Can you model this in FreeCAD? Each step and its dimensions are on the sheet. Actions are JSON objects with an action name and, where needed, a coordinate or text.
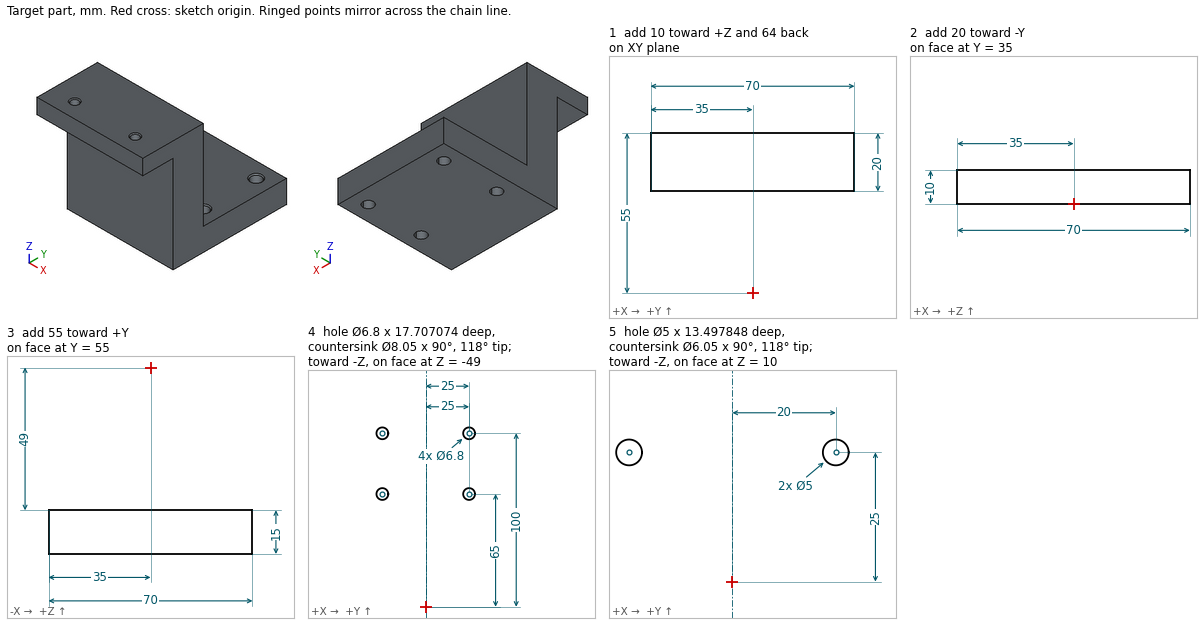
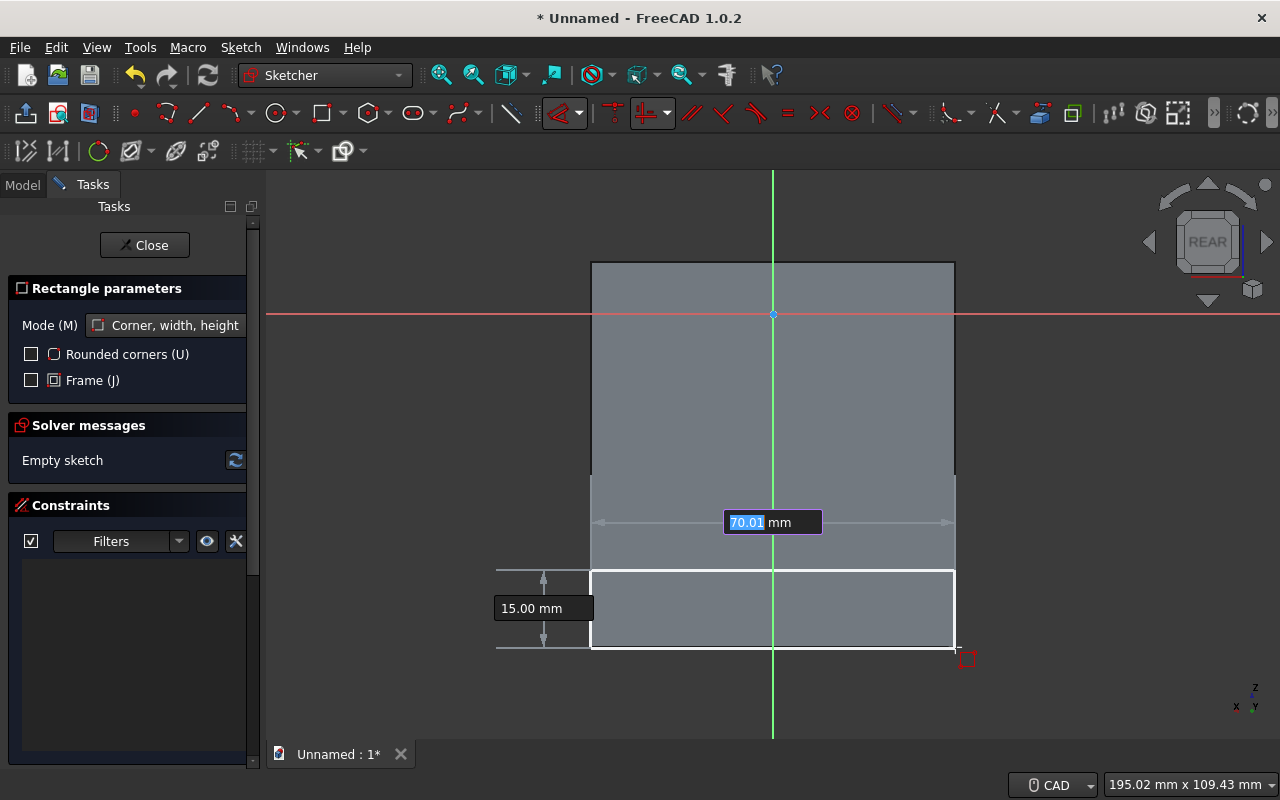
{"action": "type", "text": "70"}
{"action": "key", "text": "Tab"}
{"action": "type", "text": "15"}
{"action": "key", "text": "Return"}
{"action": "key", "text": "Escape"}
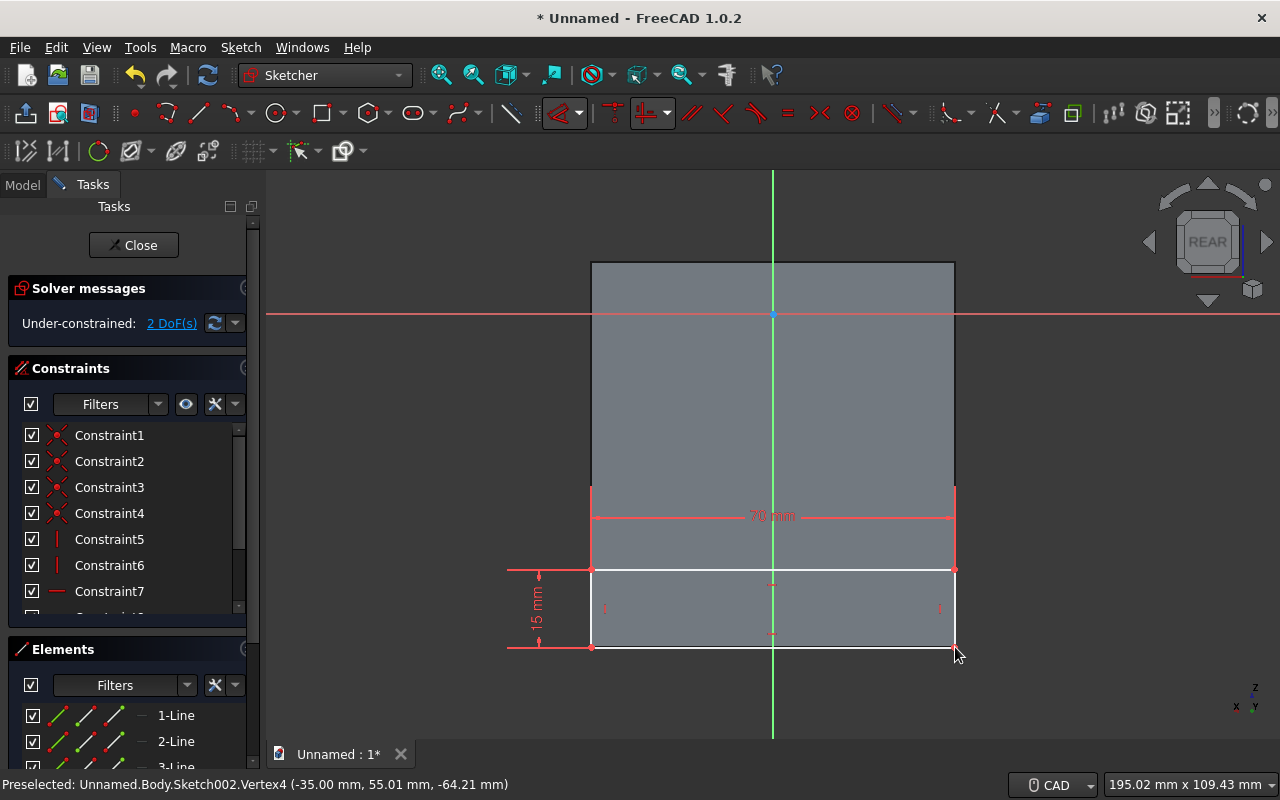
{"action": "left_click", "coordinate": [591, 570]}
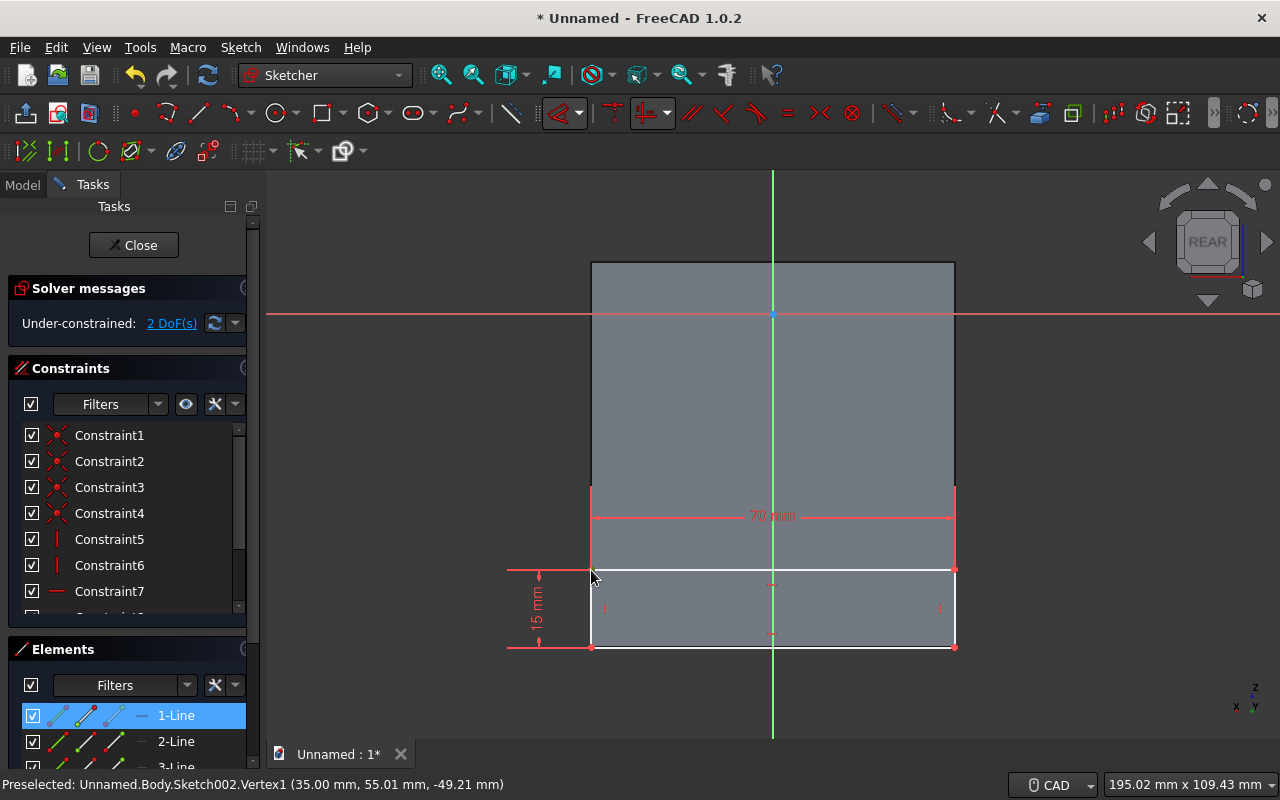
{"action": "left_click", "coordinate": [582, 114]}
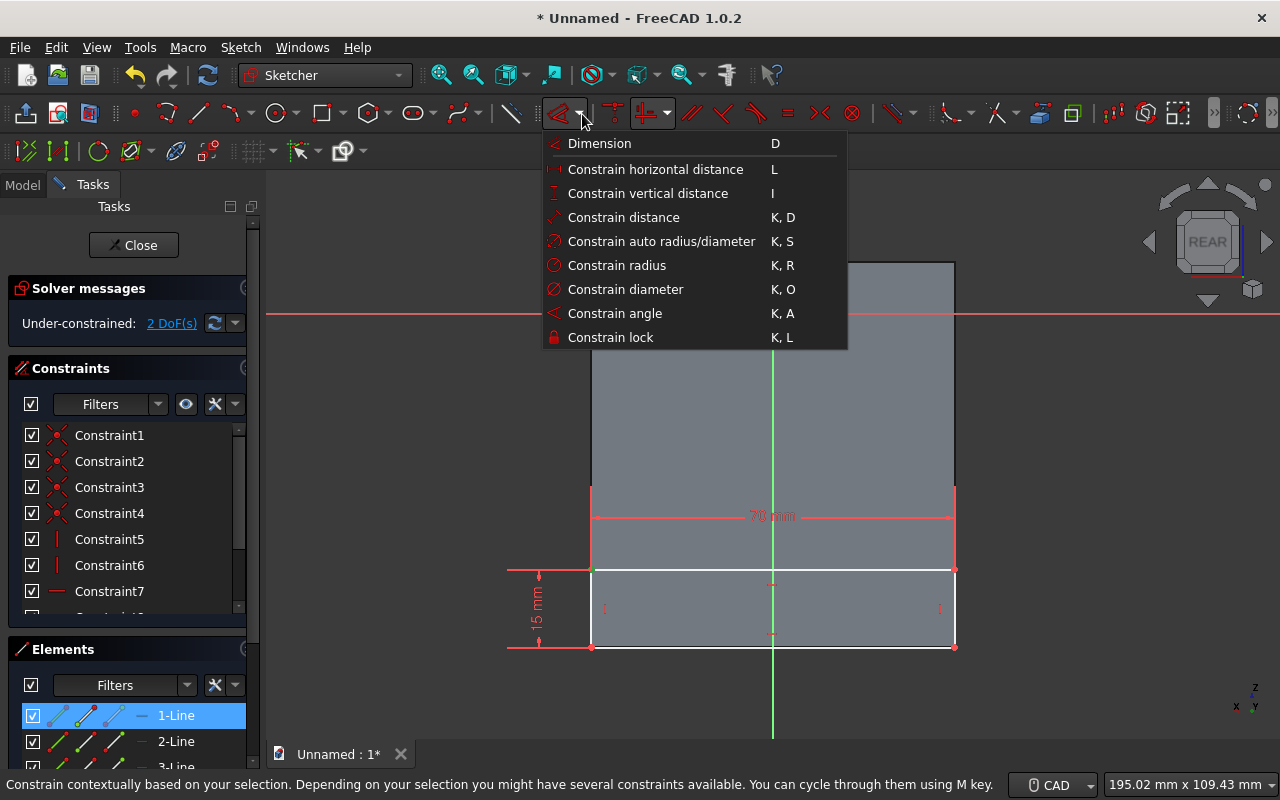
{"action": "left_click", "coordinate": [695, 169]}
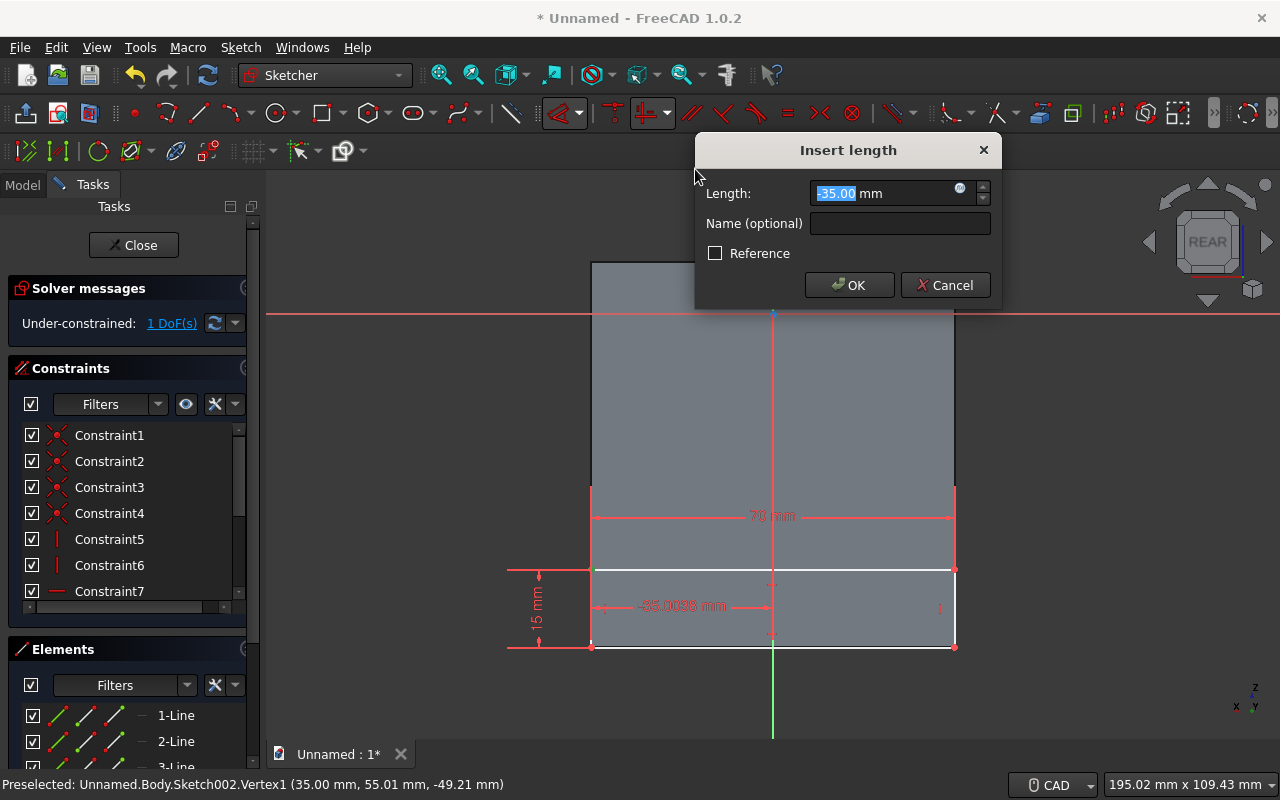
{"action": "type", "text": "-35"}
{"action": "key", "text": "Return"}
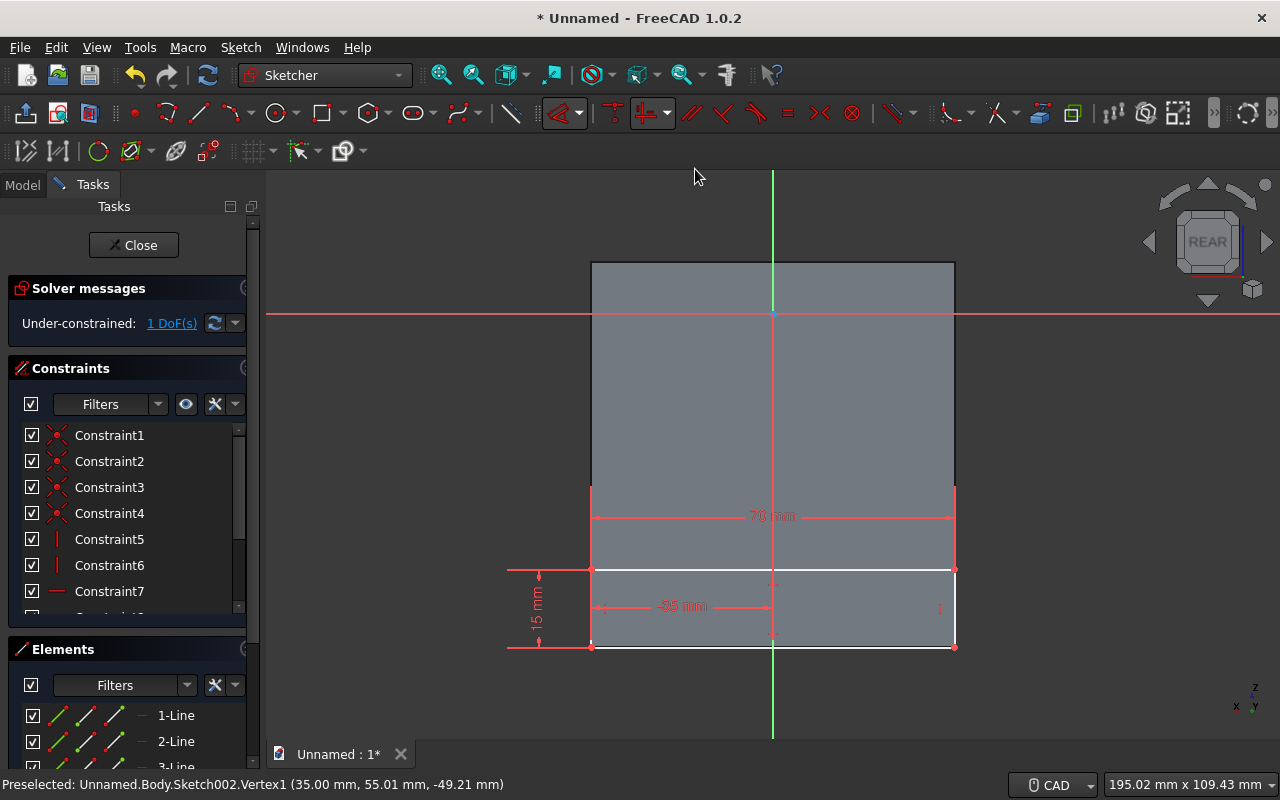
{"action": "left_click", "coordinate": [591, 570]}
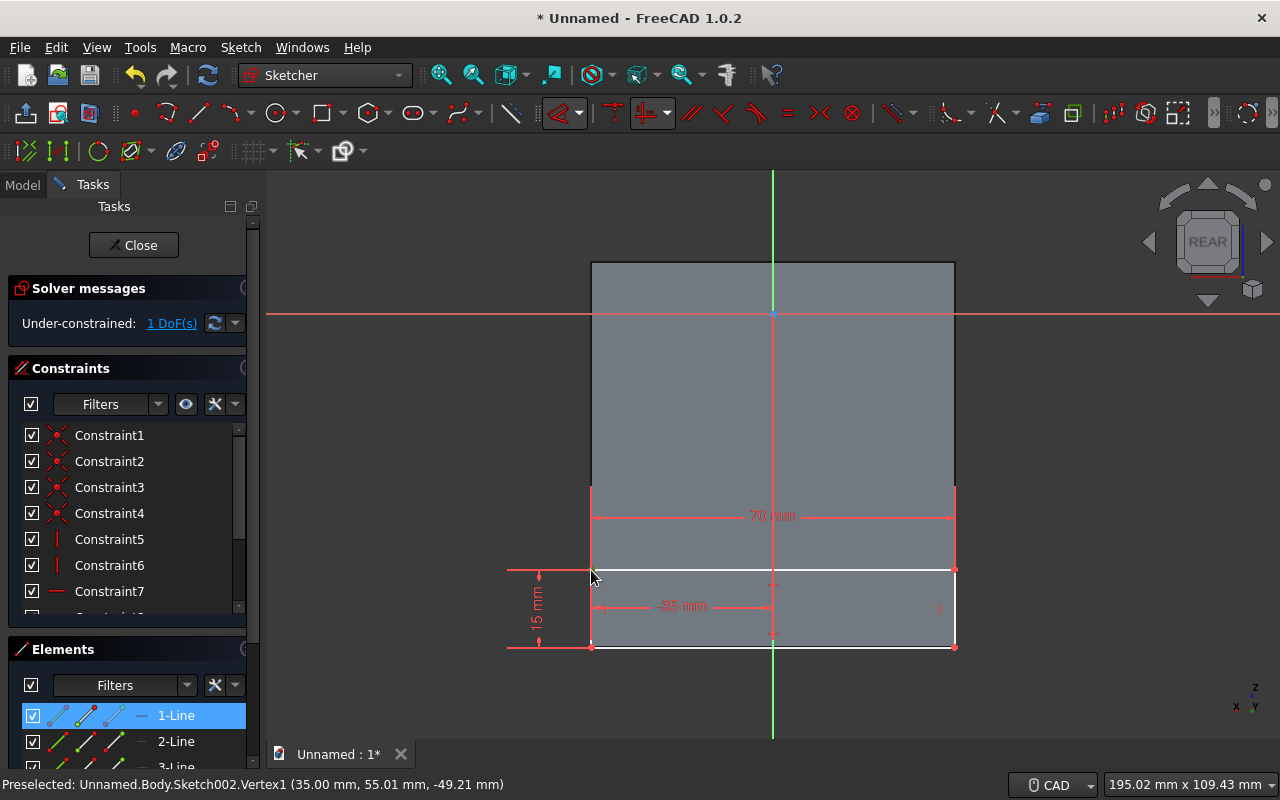
{"action": "left_click", "coordinate": [582, 114]}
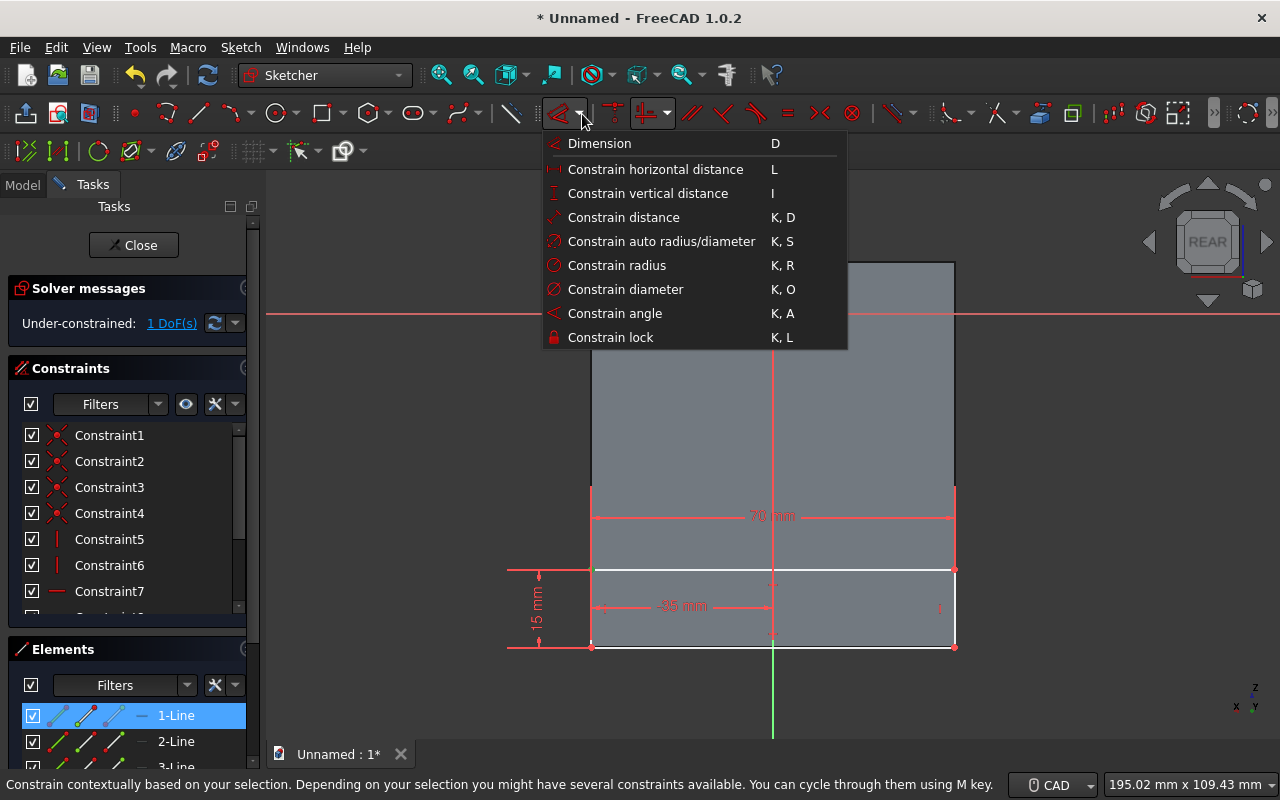
{"action": "left_click", "coordinate": [695, 193]}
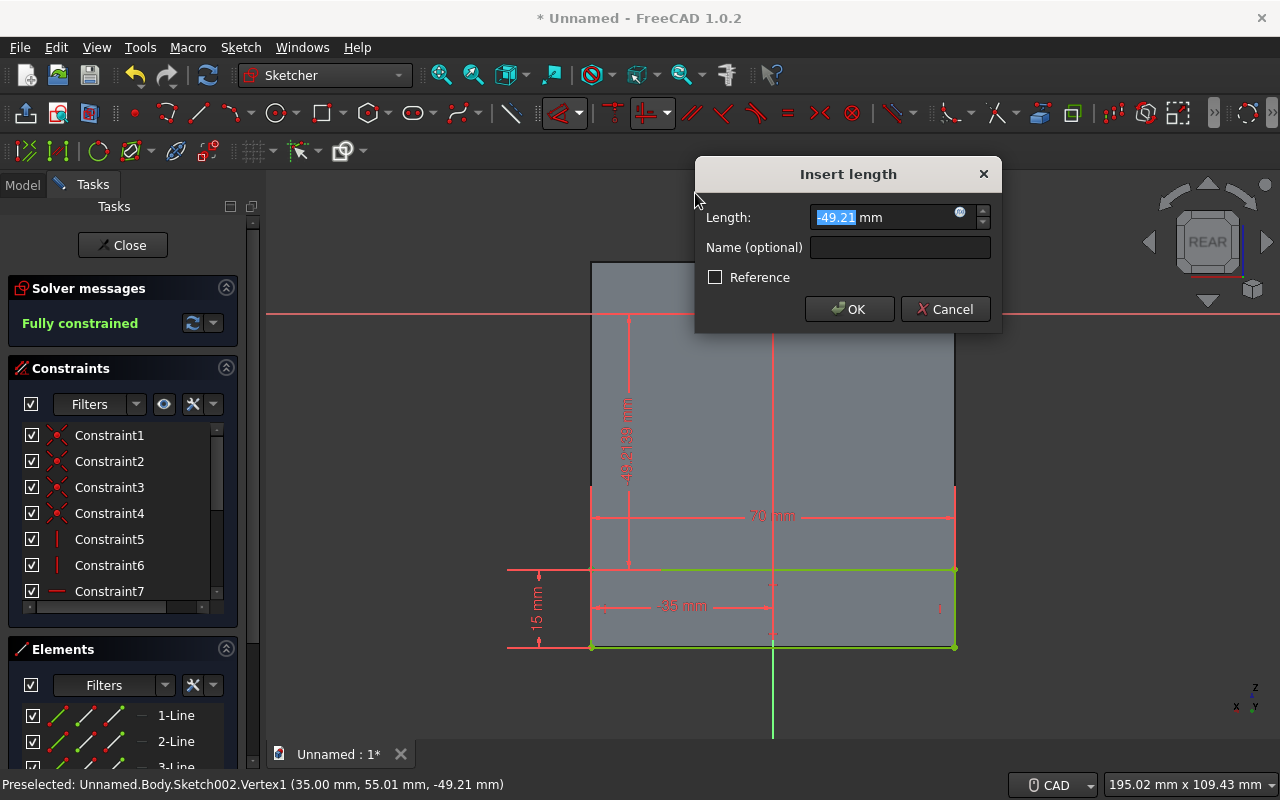
{"action": "type", "text": "-49"}
{"action": "key", "text": "Return"}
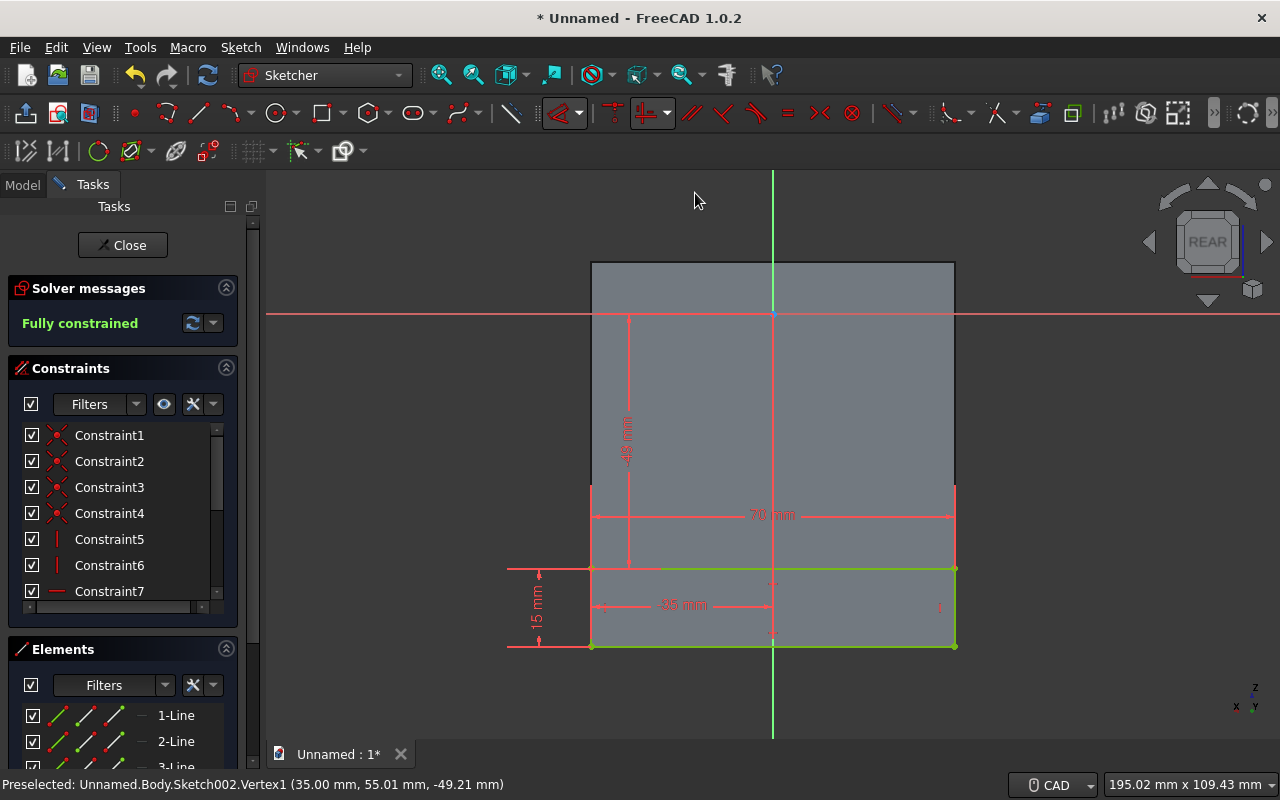
{"action": "left_click", "coordinate": [123, 245]}